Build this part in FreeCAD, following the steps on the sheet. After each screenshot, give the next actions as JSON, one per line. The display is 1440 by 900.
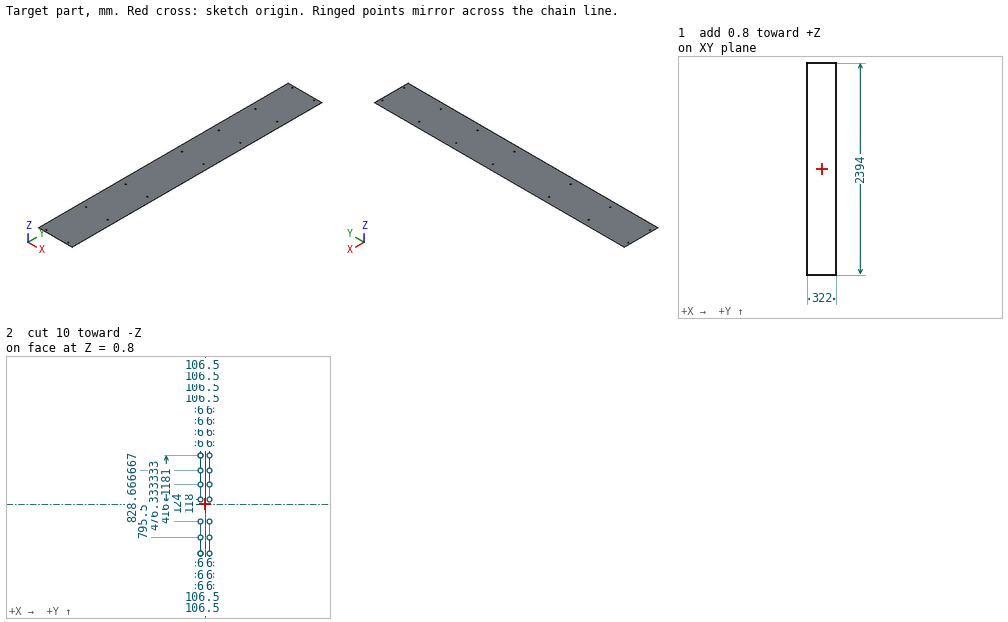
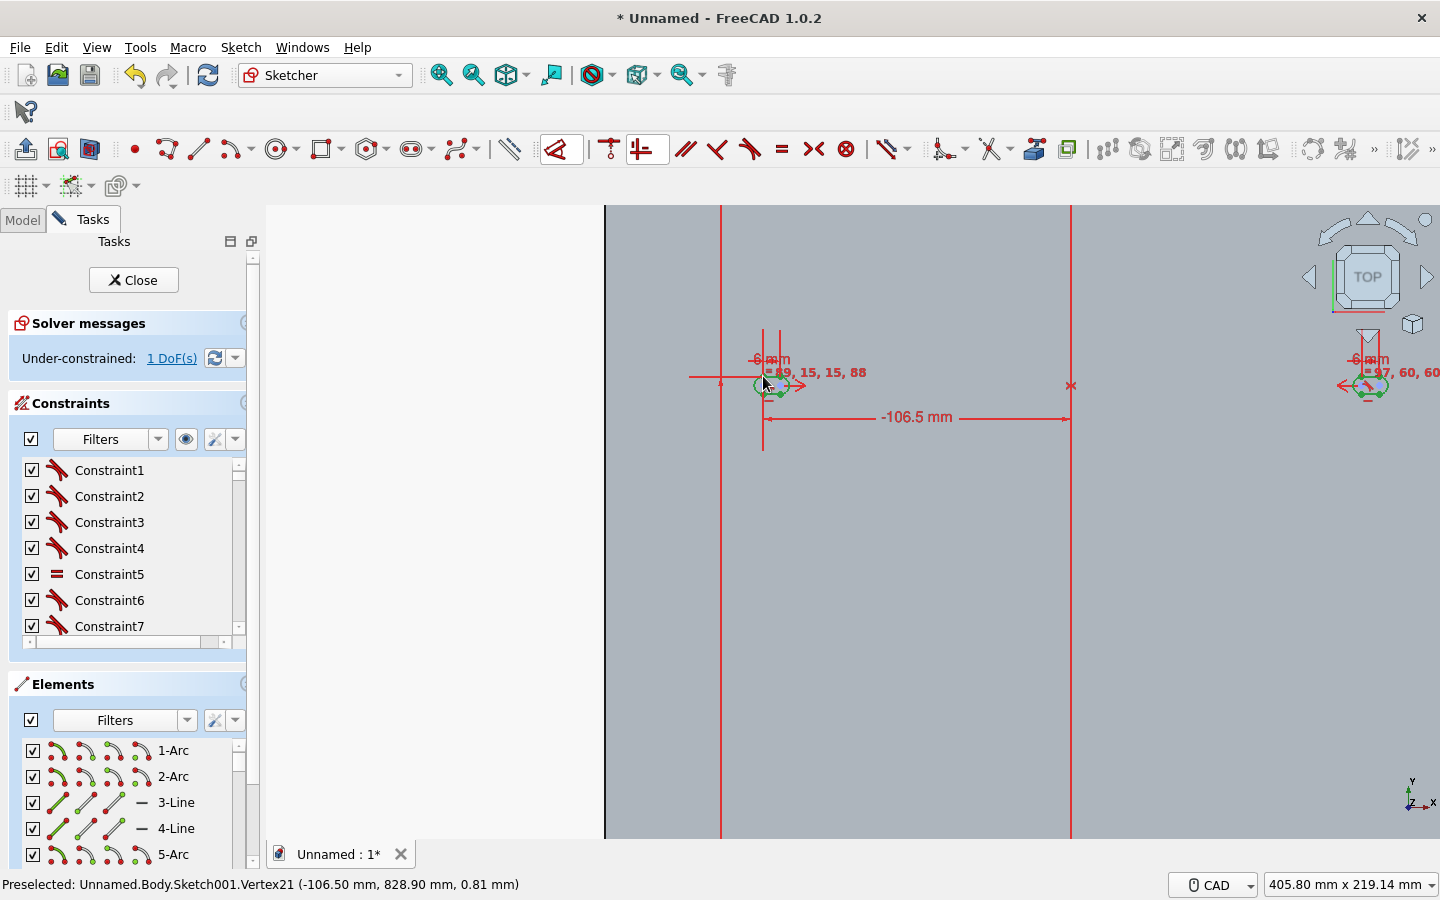
{"action": "scroll", "coordinate": [766, 376], "scroll_direction": "down", "scroll_amount": 14}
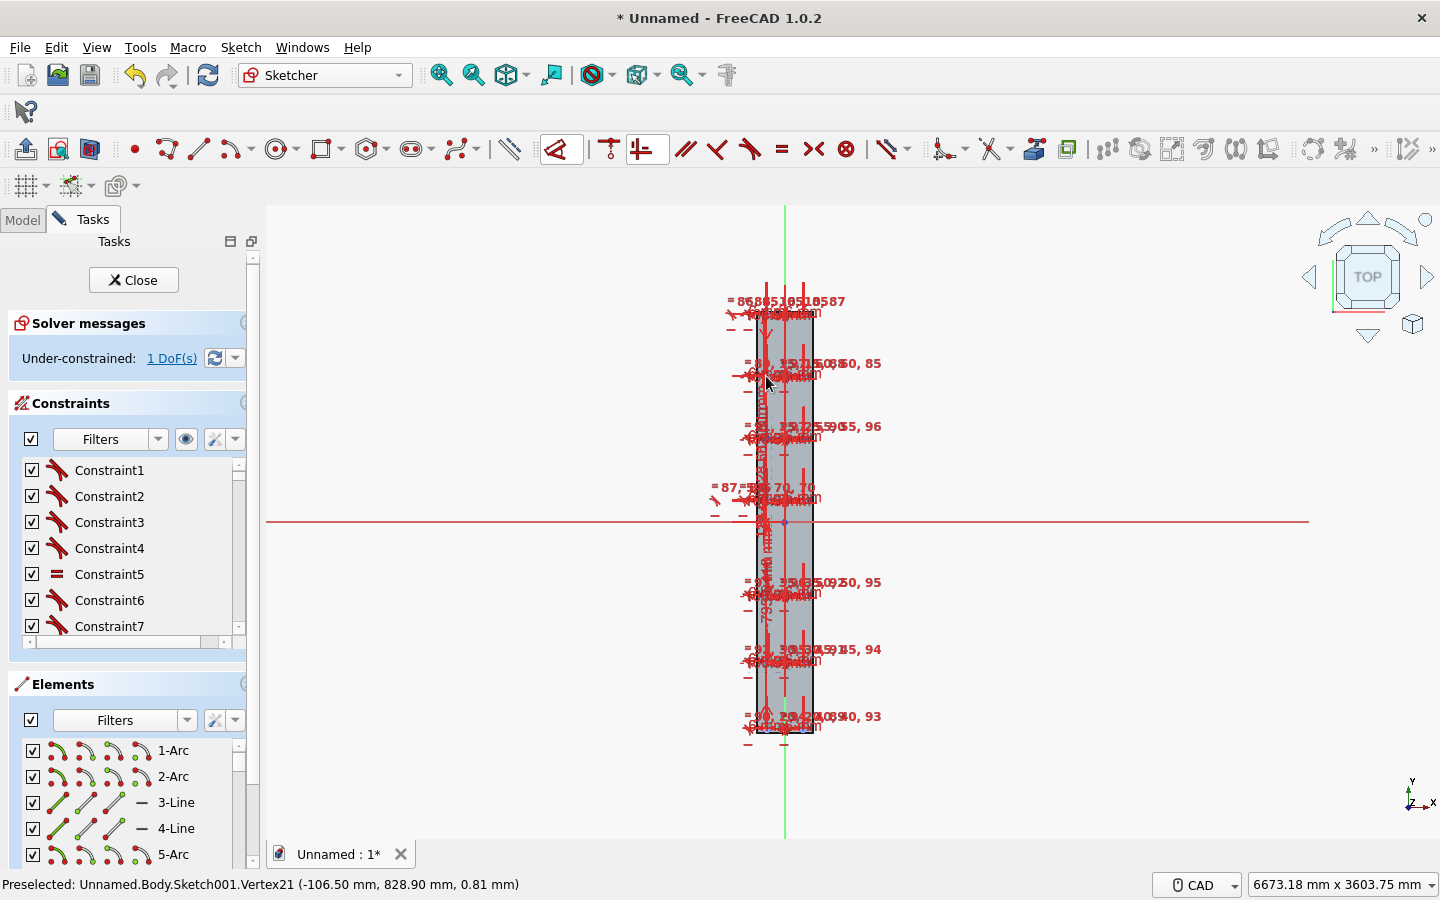
{"action": "scroll", "coordinate": [766, 439], "scroll_direction": "up", "scroll_amount": 14}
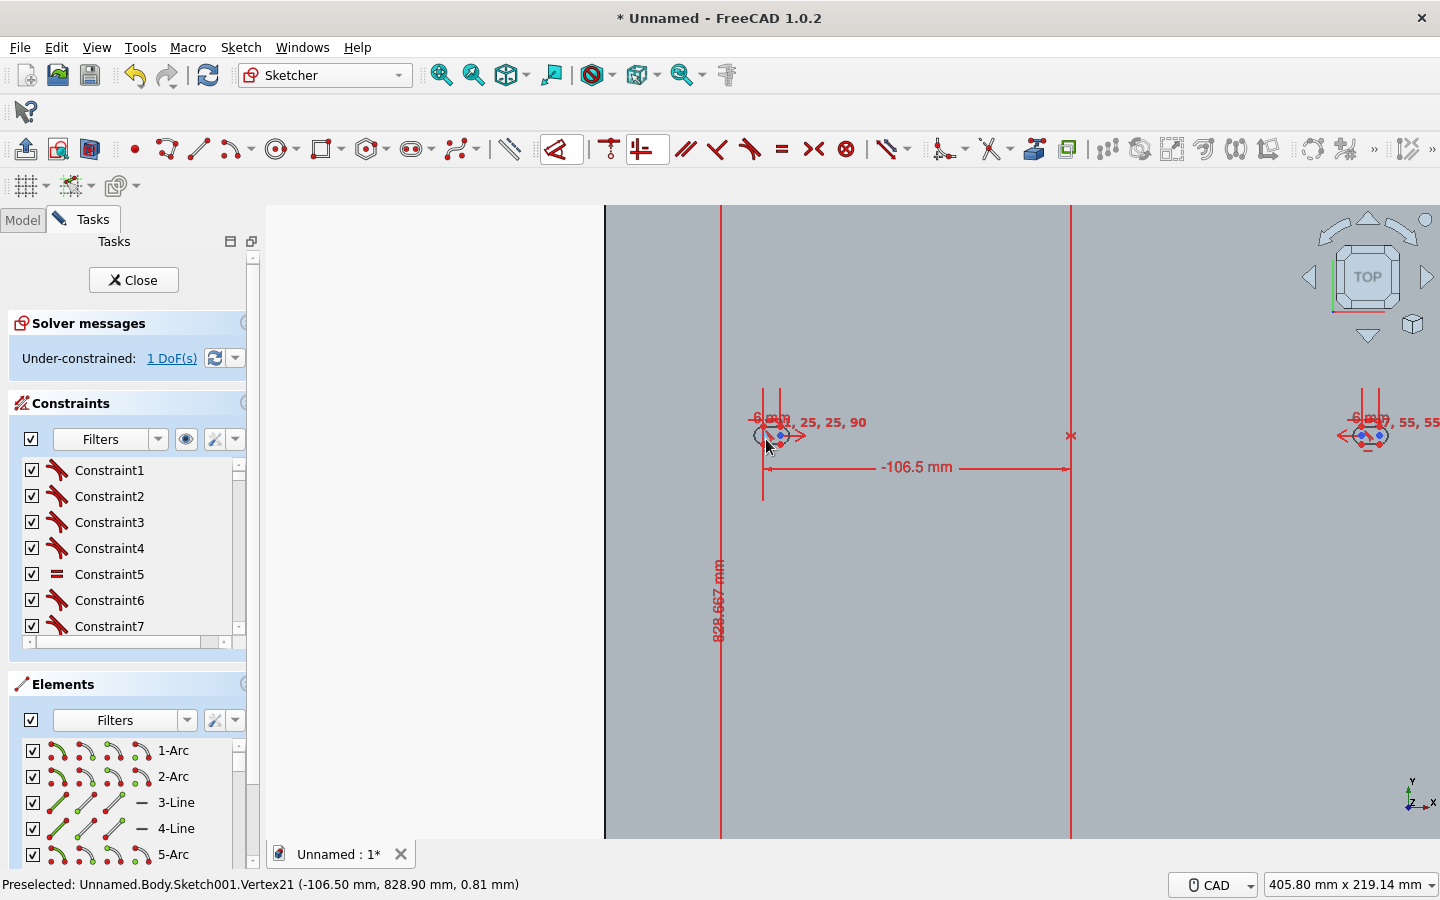
{"action": "left_click", "coordinate": [763, 427]}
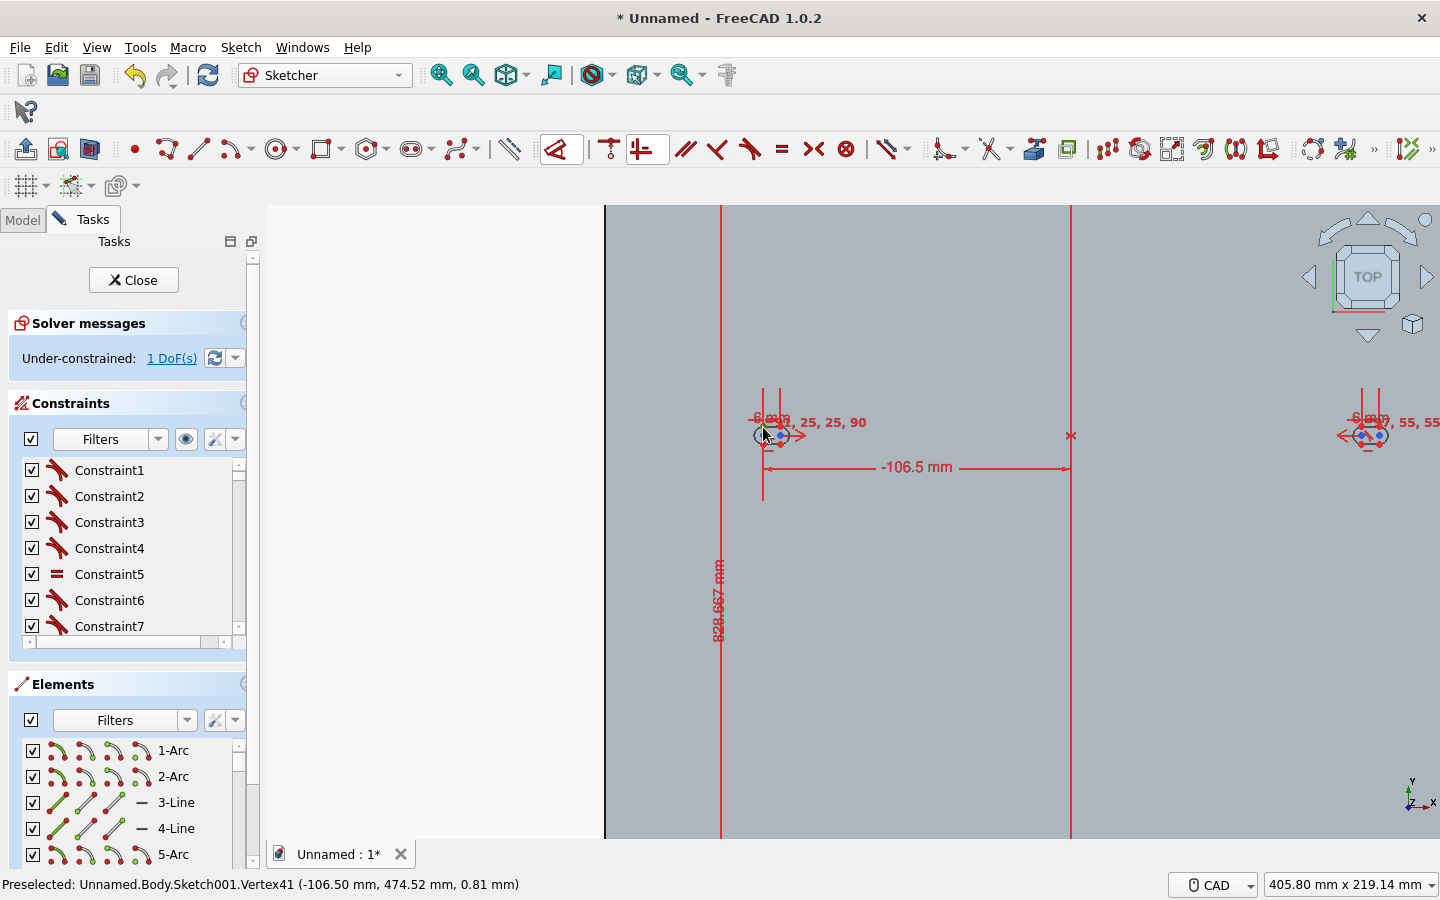
{"action": "key", "text": "i"}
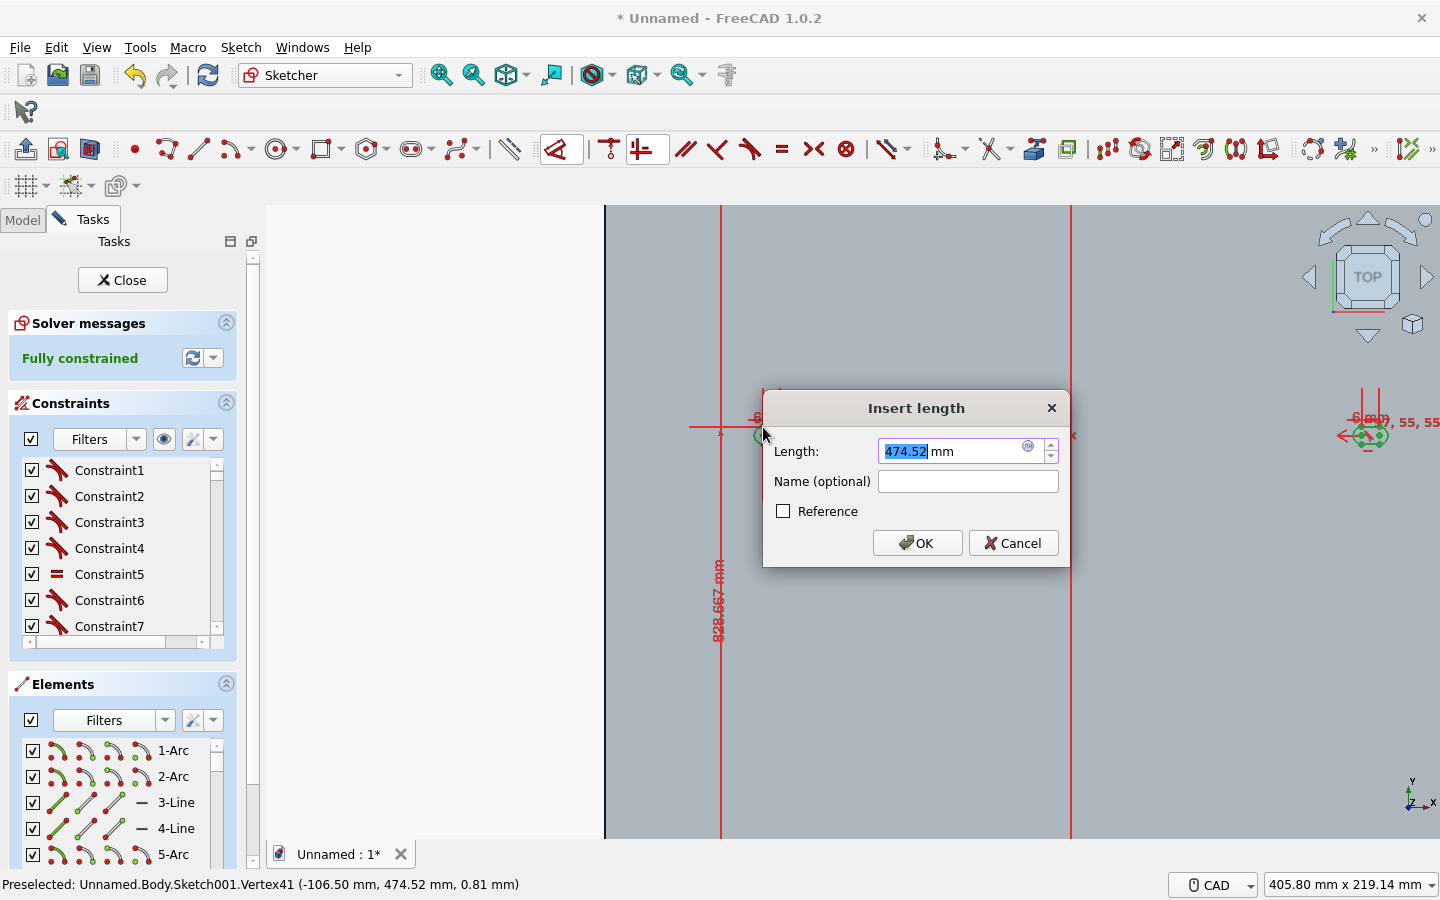
{"action": "type", "text": "476.333333"}
{"action": "key", "text": "Return"}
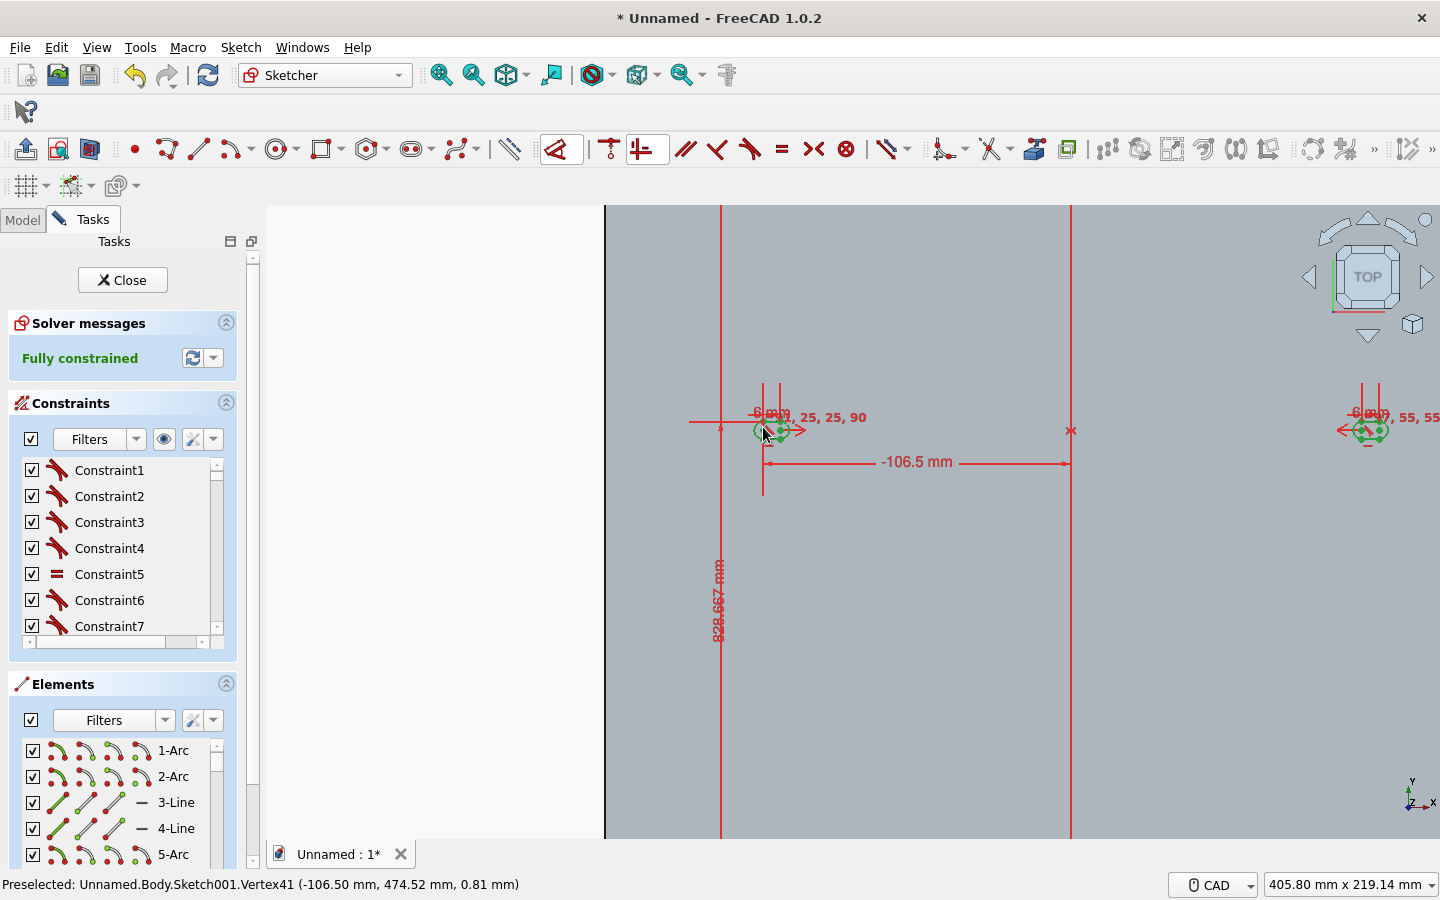
{"action": "left_click", "coordinate": [123, 280]}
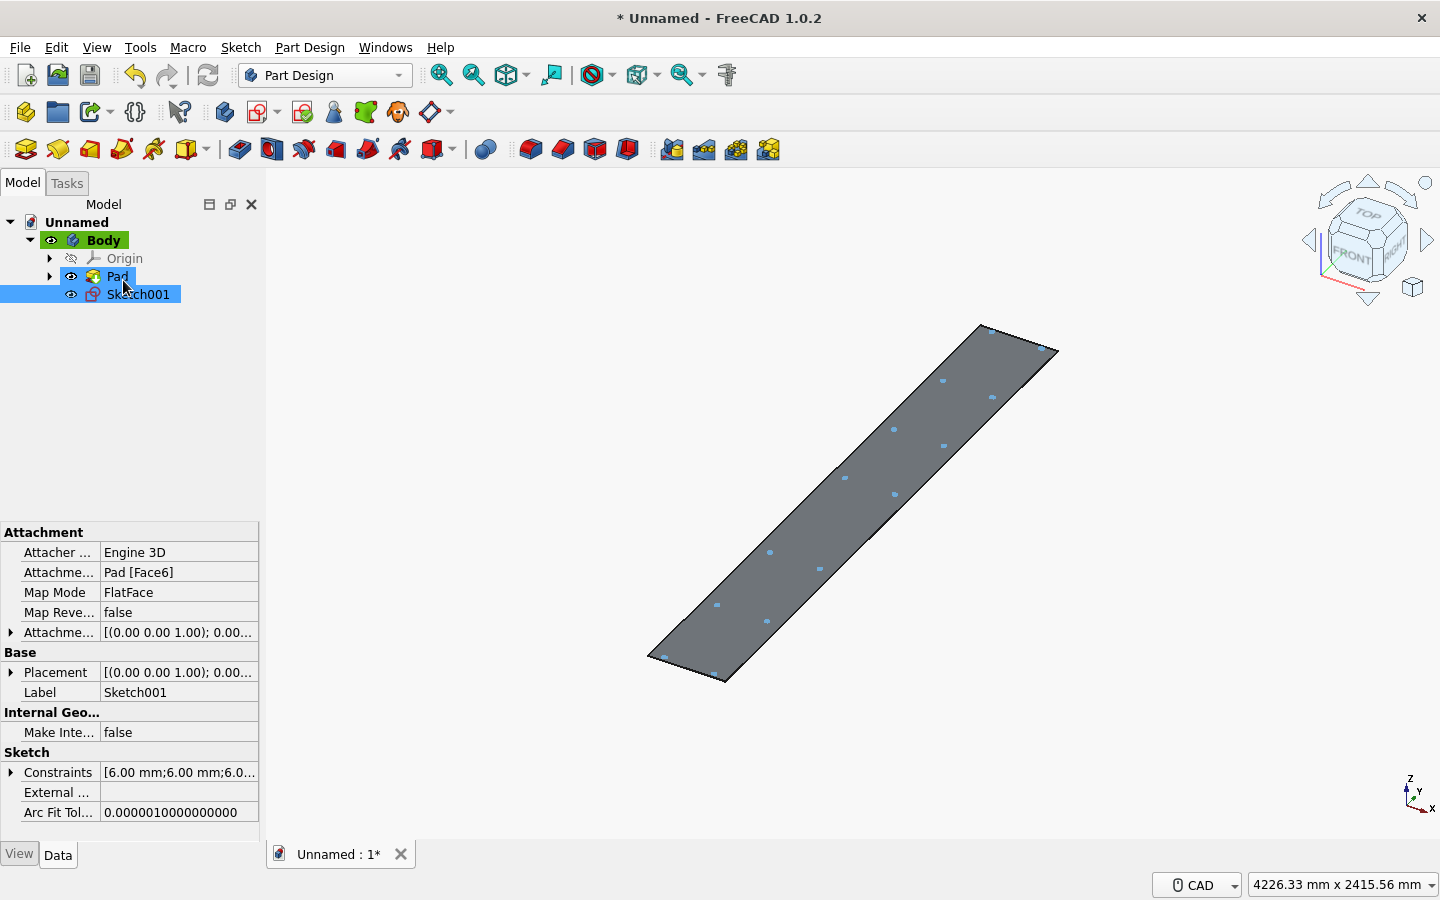
{"action": "left_click", "coordinate": [240, 150]}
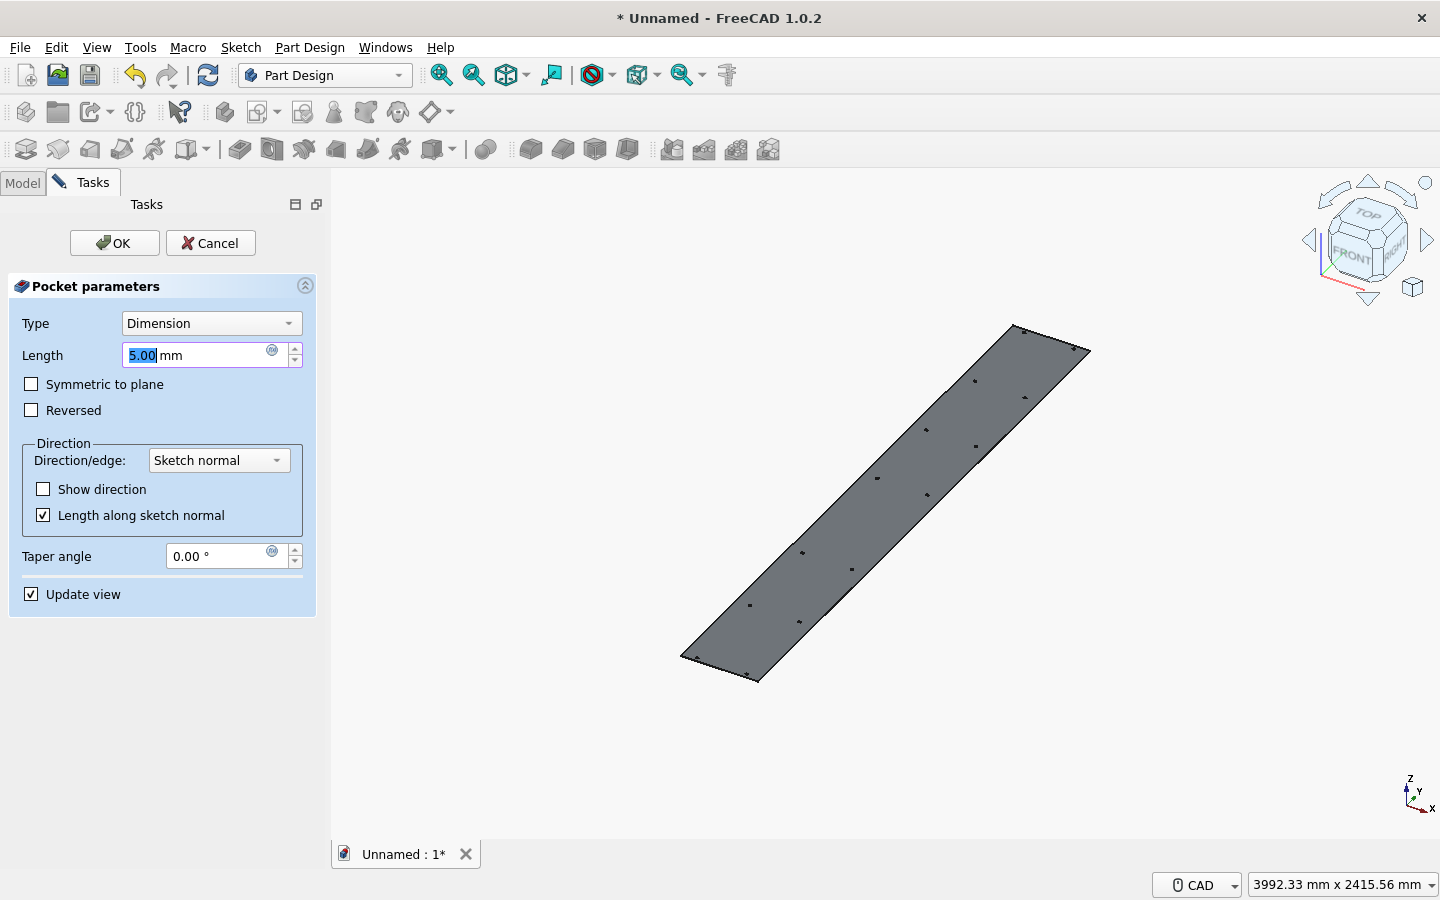
{"action": "type", "text": "10"}
{"action": "key", "text": "Tab"}